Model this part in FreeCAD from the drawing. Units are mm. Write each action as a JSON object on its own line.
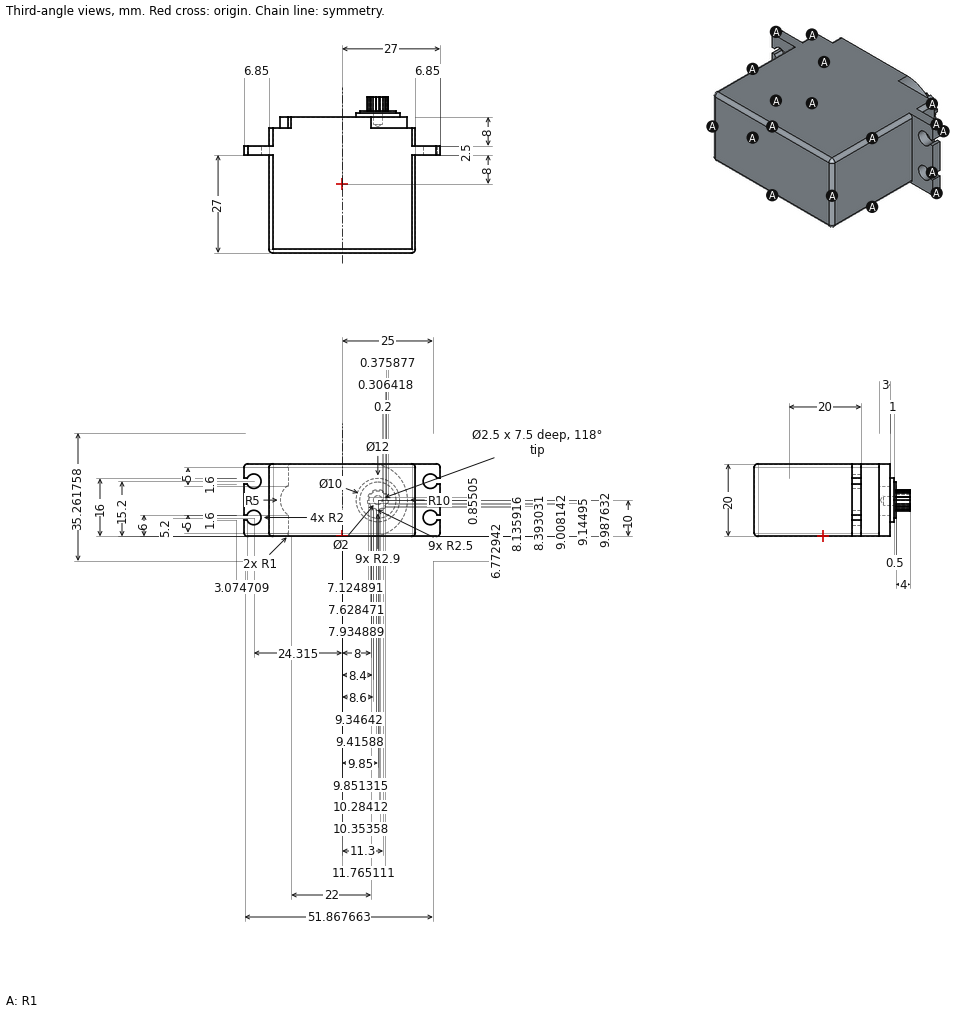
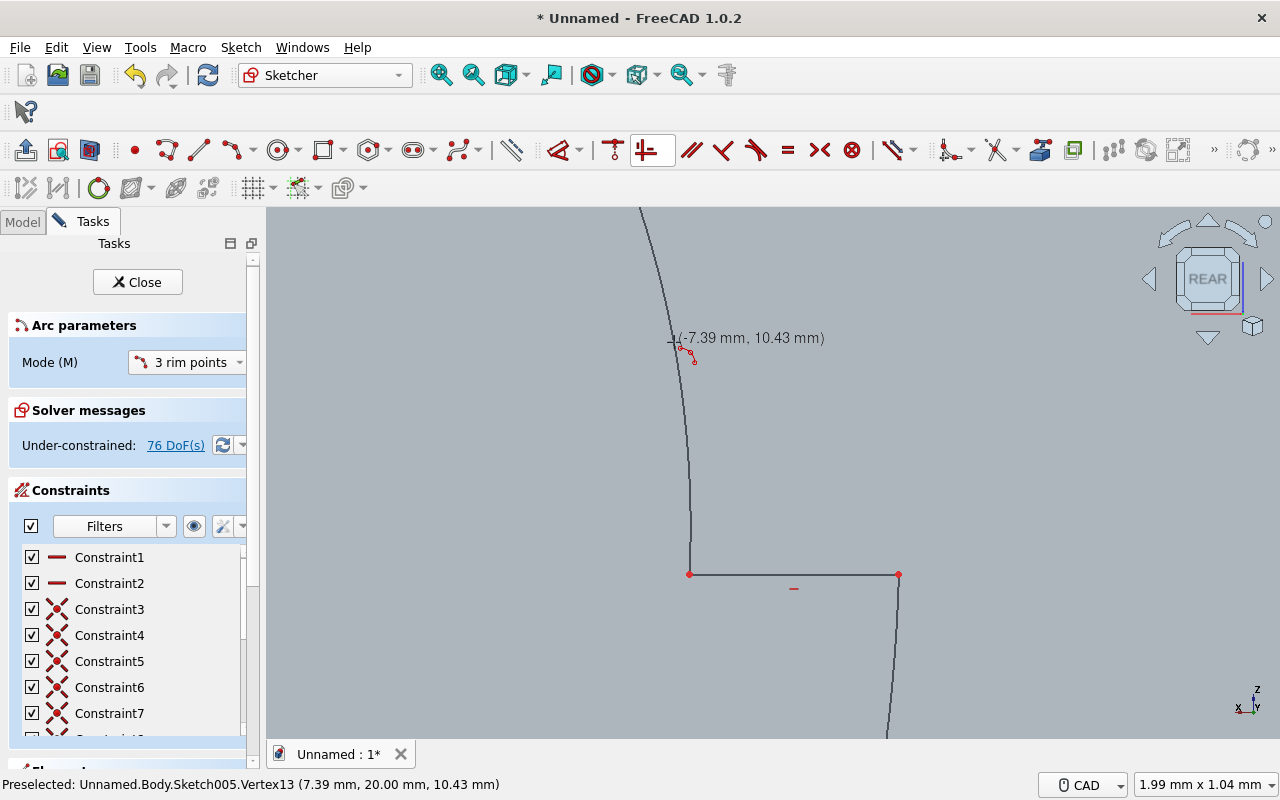
{"action": "scroll", "coordinate": [679, 373], "scroll_direction": "down", "scroll_amount": 15}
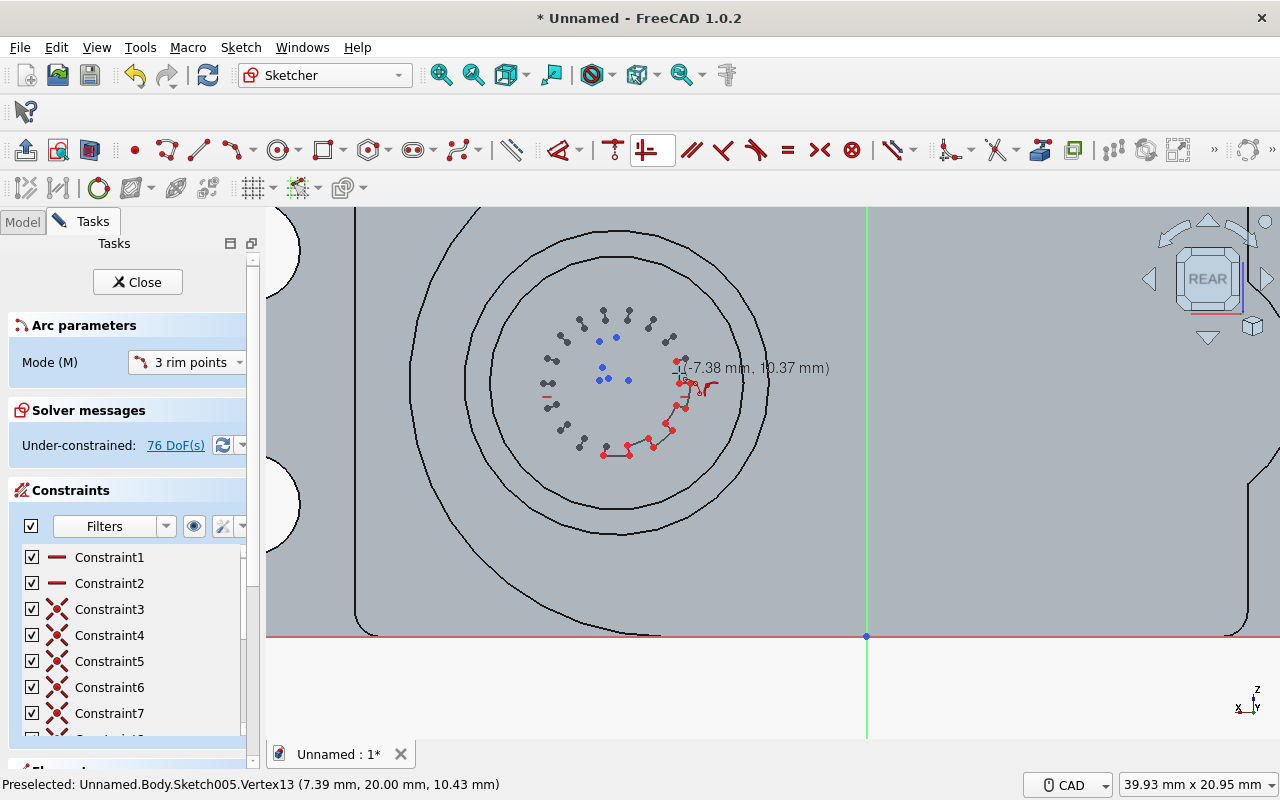
{"action": "scroll", "coordinate": [686, 358], "scroll_direction": "up", "scroll_amount": 6}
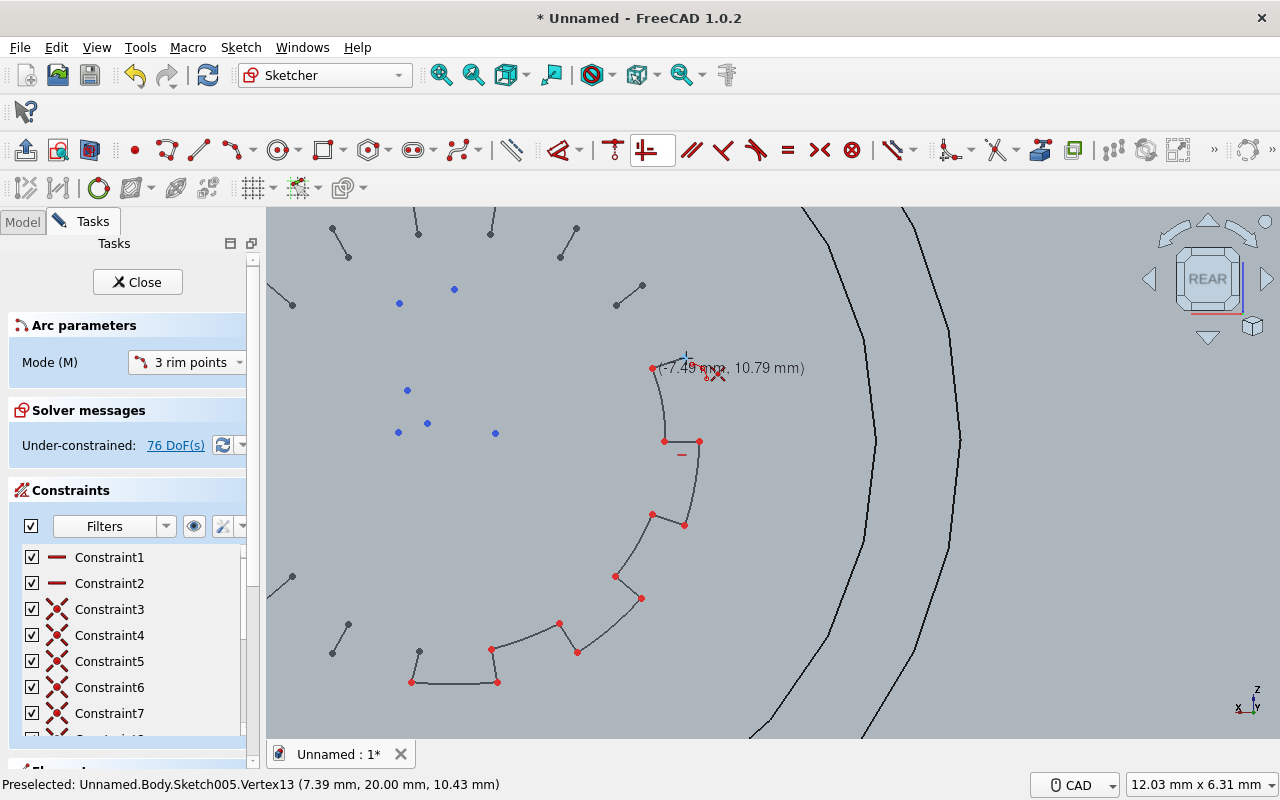
{"action": "left_click", "coordinate": [685, 358]}
{"action": "left_click", "coordinate": [643, 285]}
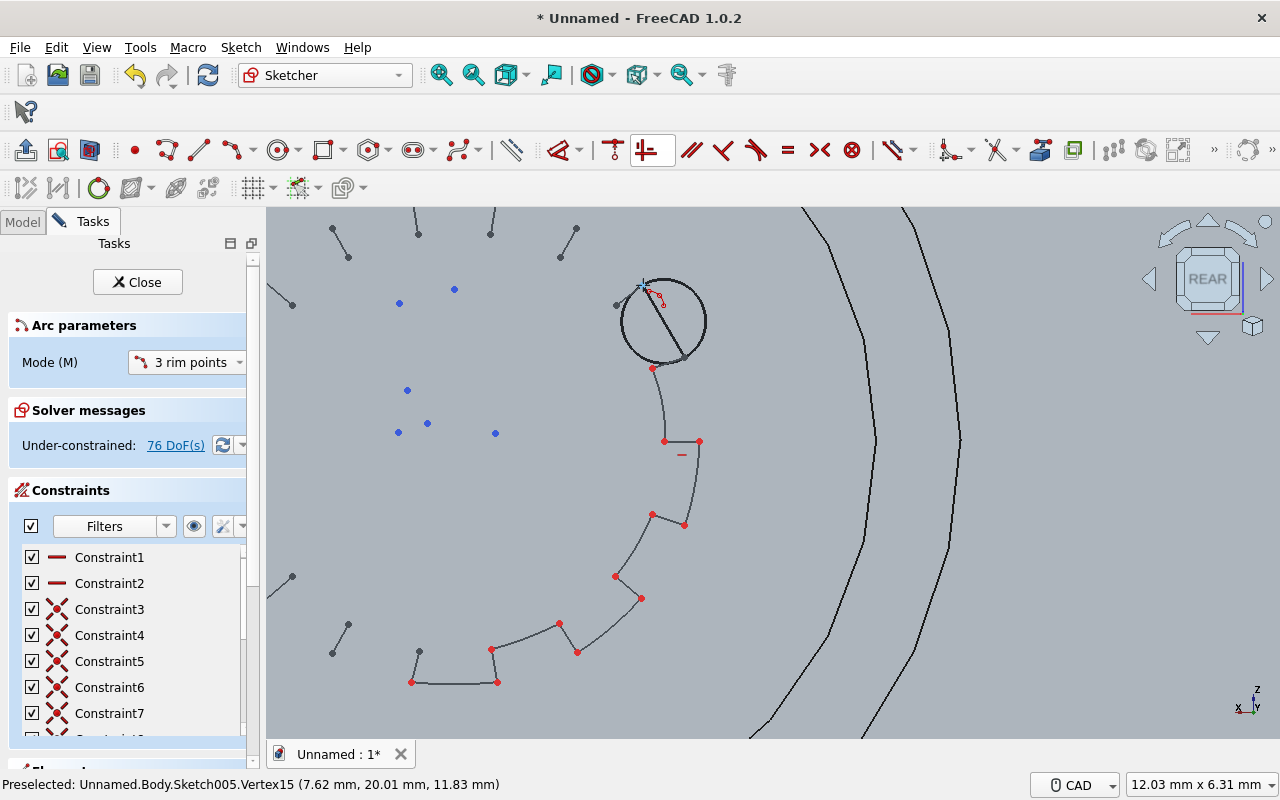
{"action": "scroll", "coordinate": [666, 317], "scroll_direction": "up", "scroll_amount": 8}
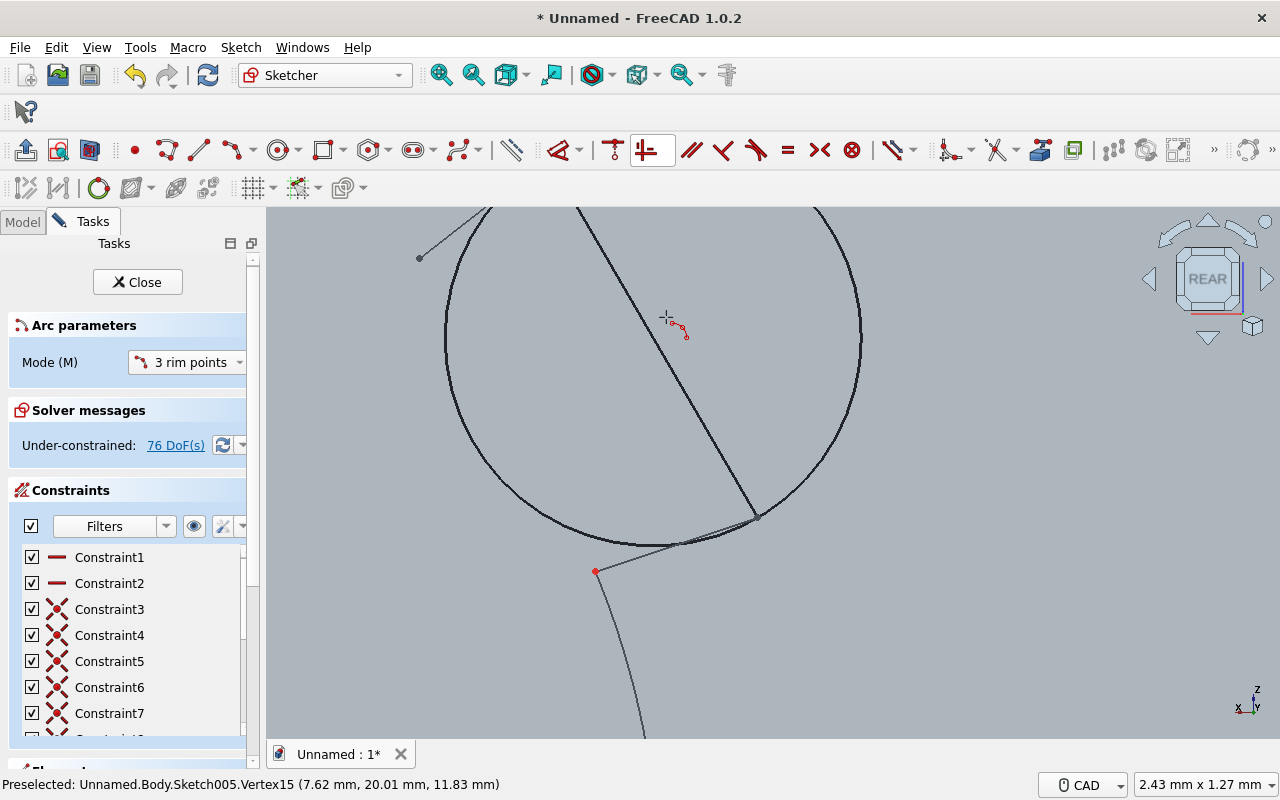
{"action": "left_click", "coordinate": [666, 318]}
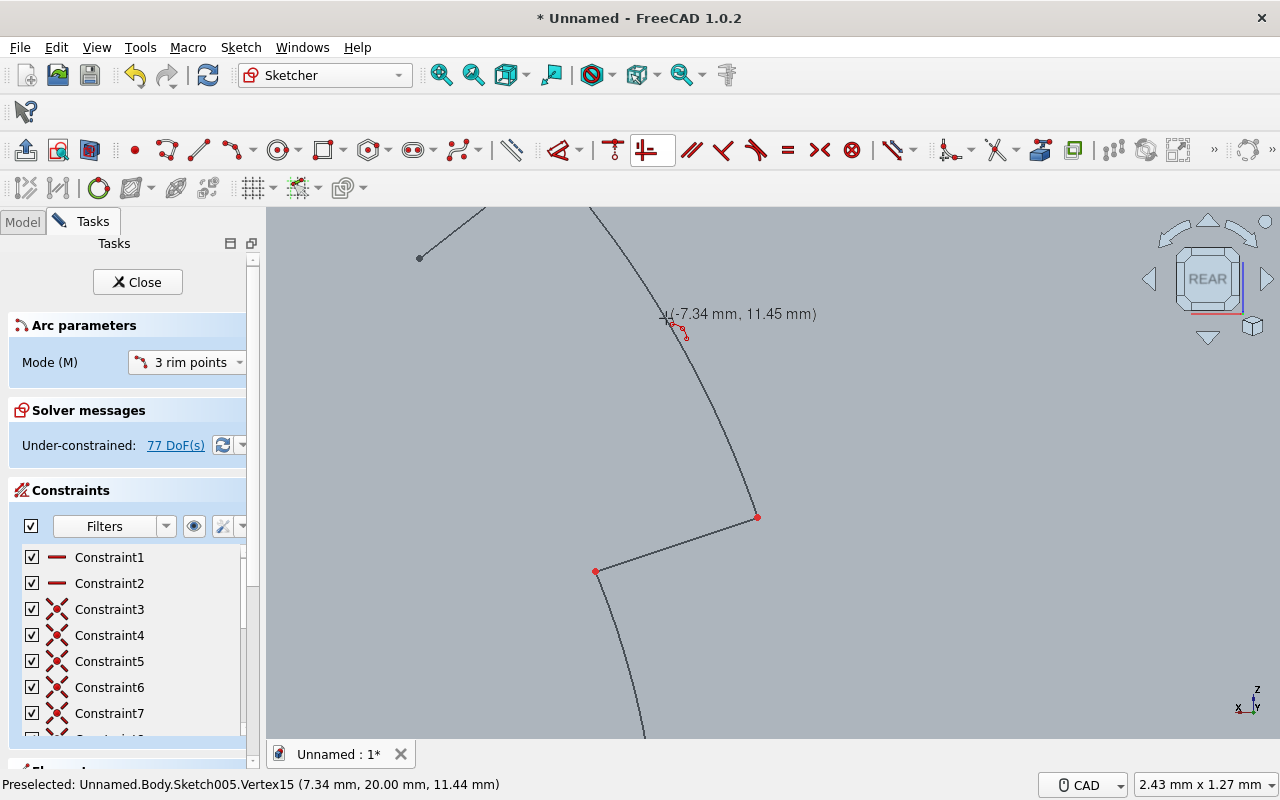
{"action": "scroll", "coordinate": [681, 347], "scroll_direction": "down", "scroll_amount": 14}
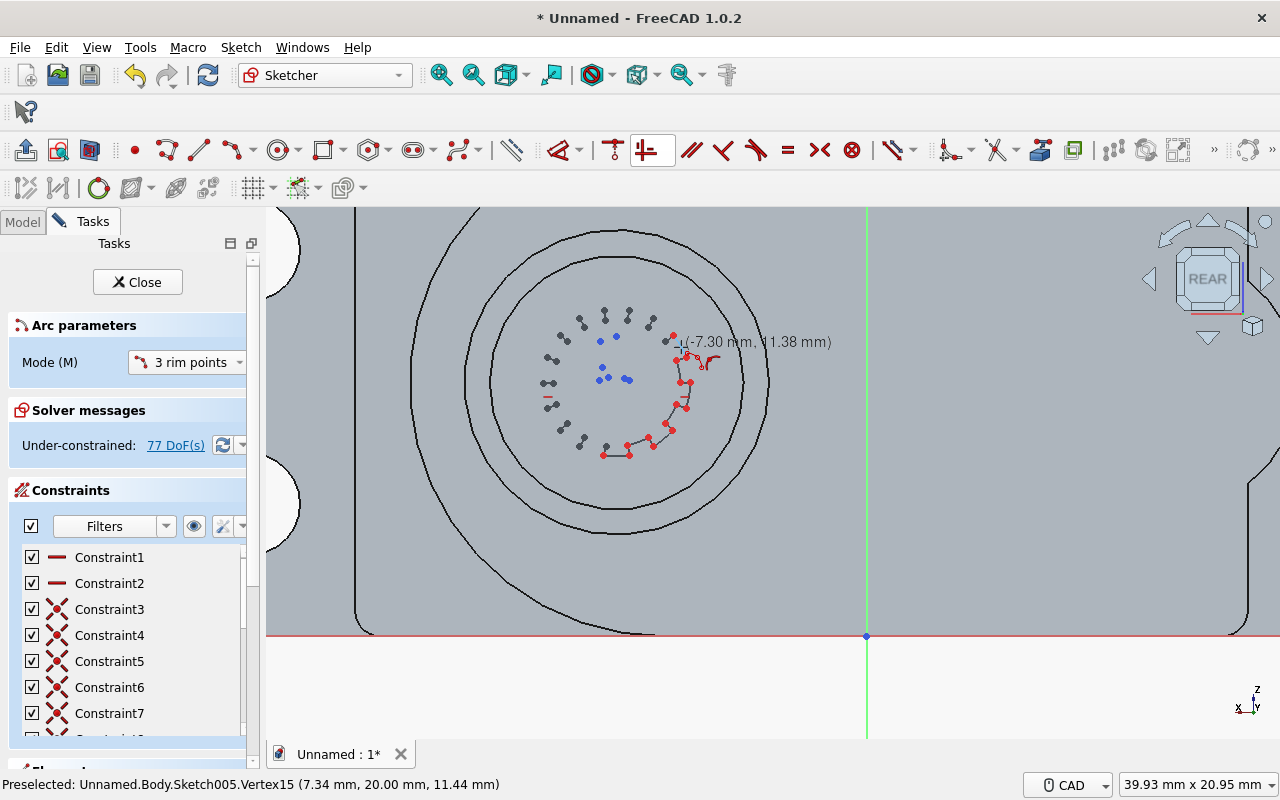
{"action": "scroll", "coordinate": [665, 341], "scroll_direction": "up", "scroll_amount": 6}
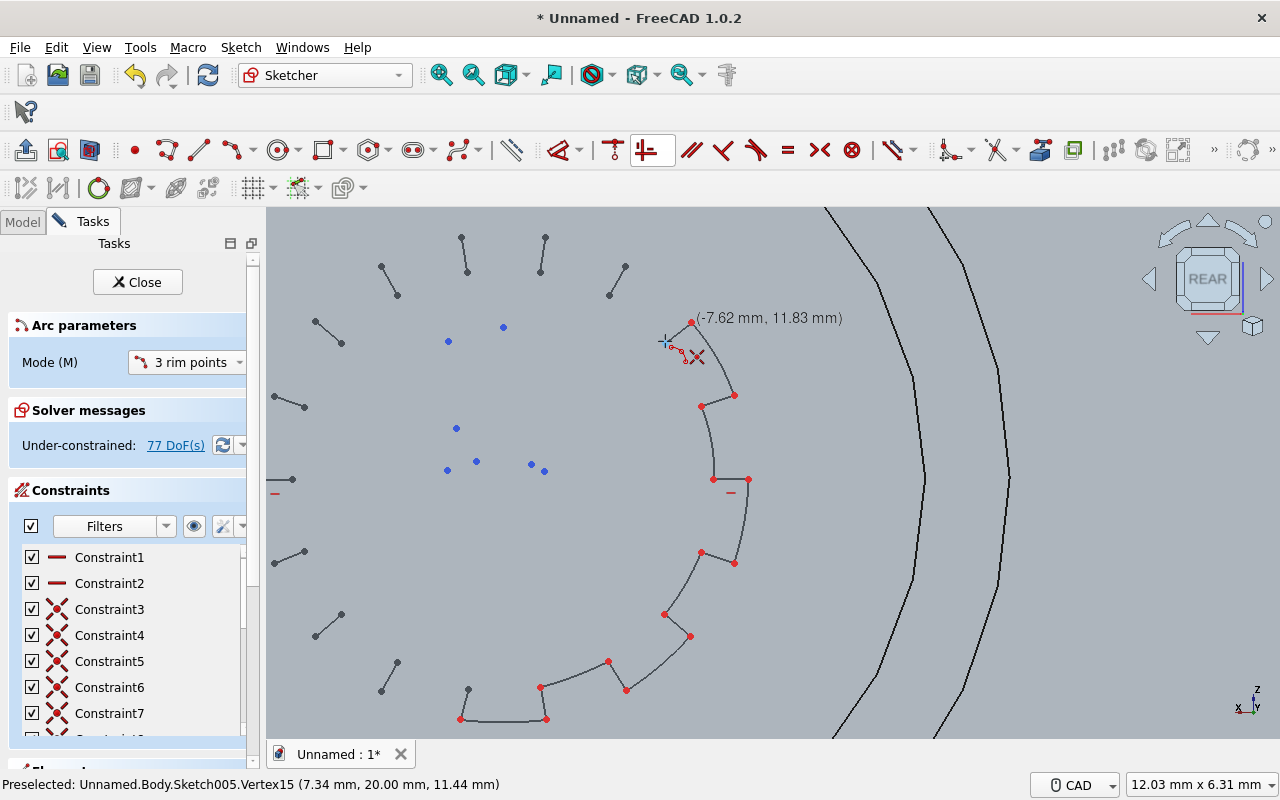
{"action": "left_click", "coordinate": [666, 343]}
{"action": "left_click", "coordinate": [609, 296]}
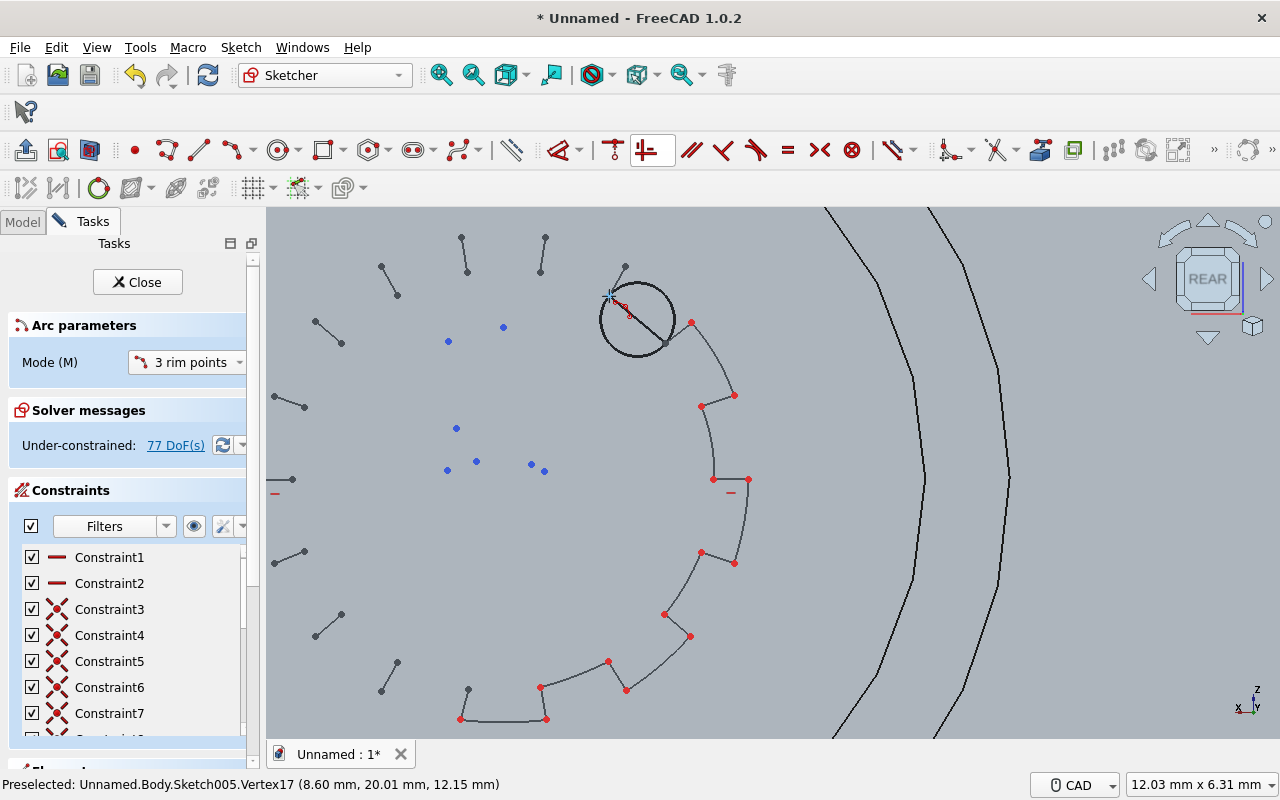
{"action": "scroll", "coordinate": [639, 316], "scroll_direction": "up", "scroll_amount": 9}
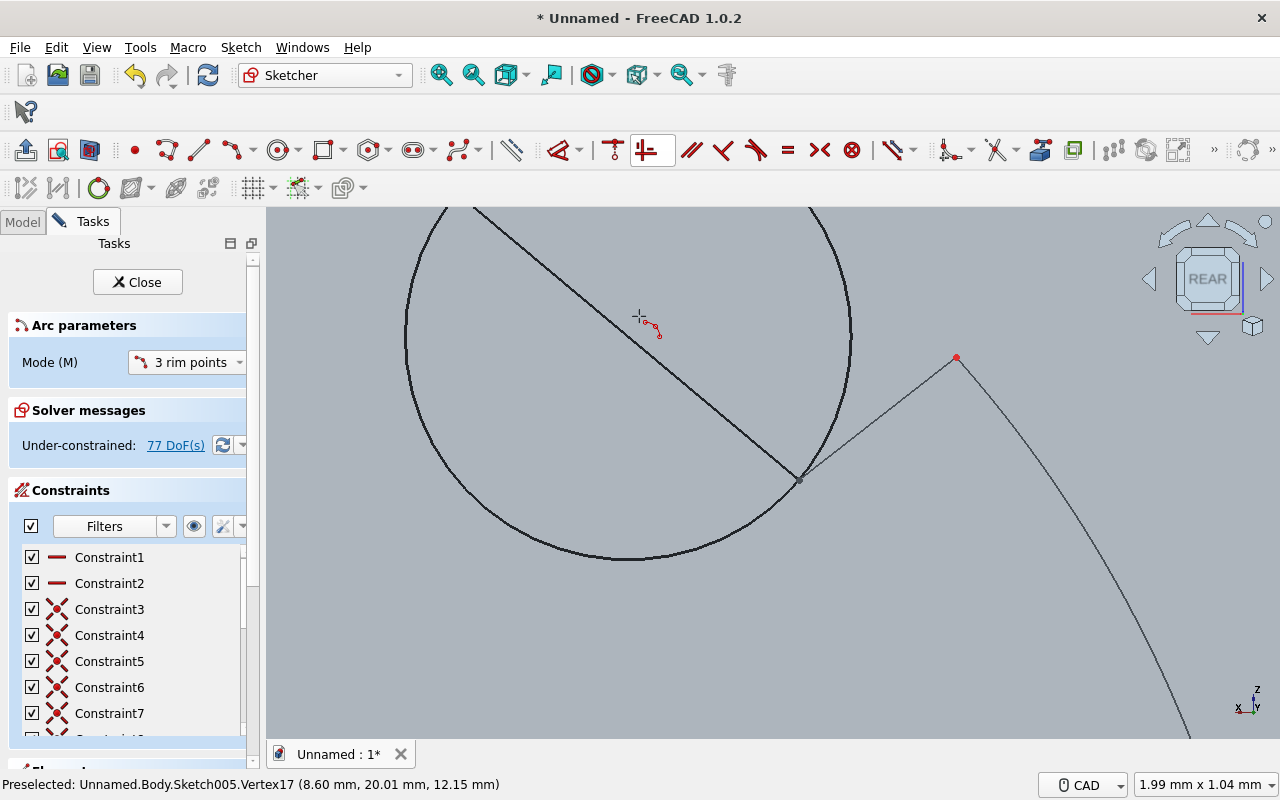
{"action": "left_click", "coordinate": [639, 315]}